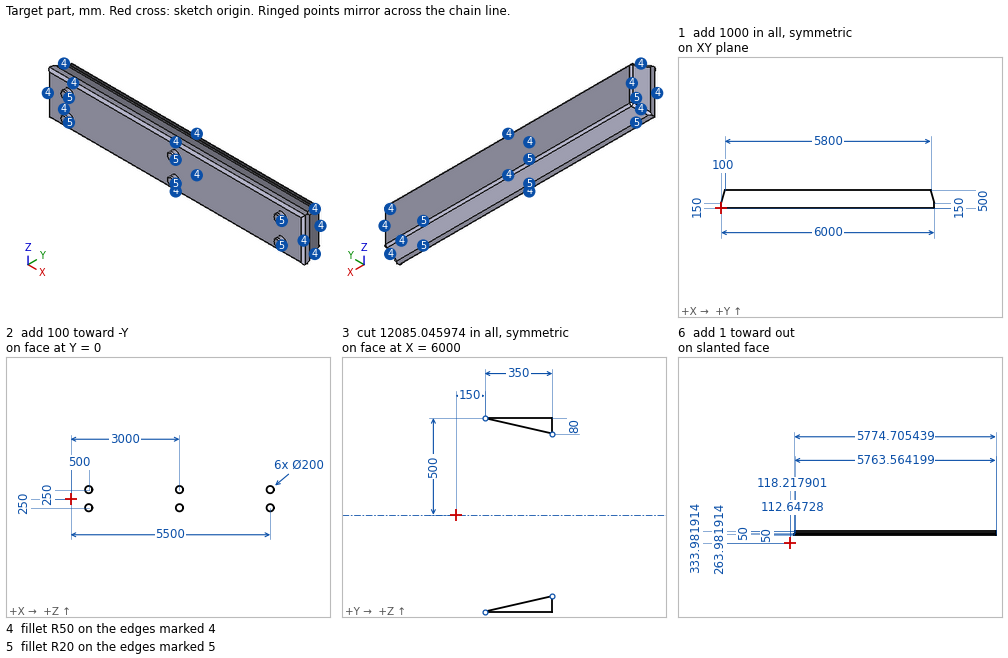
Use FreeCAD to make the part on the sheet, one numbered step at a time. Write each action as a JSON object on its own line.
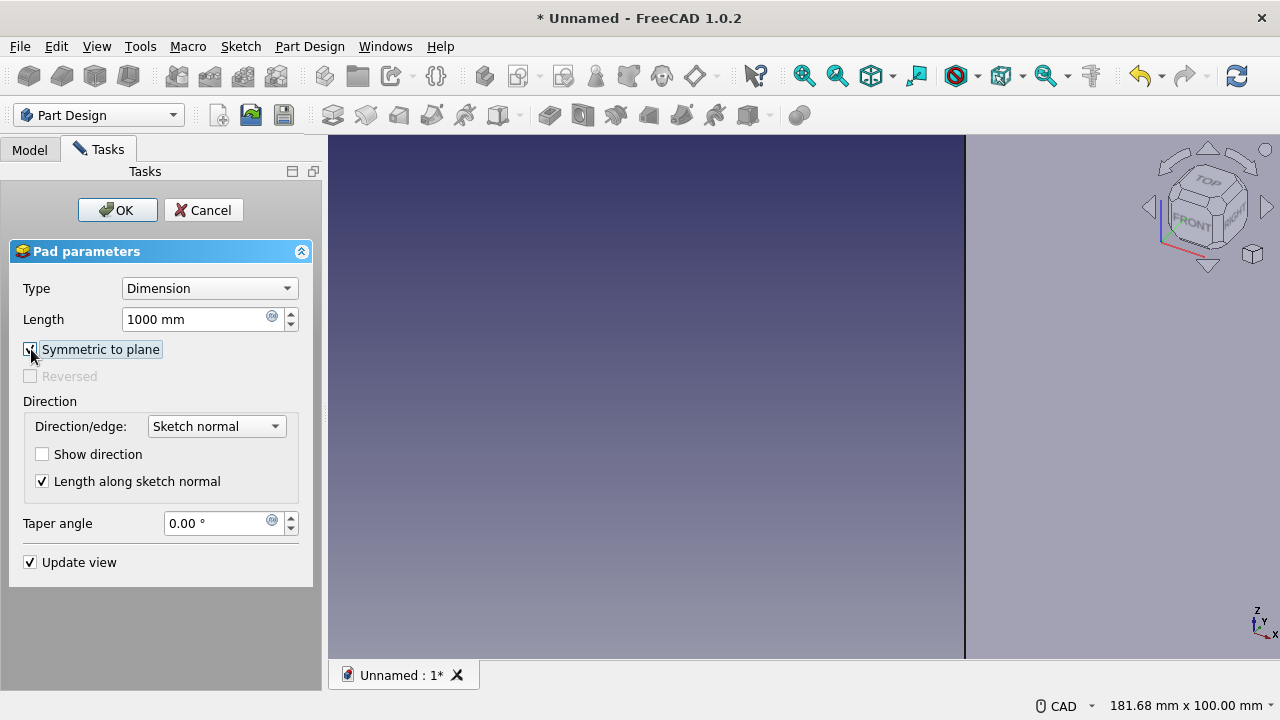
{"action": "left_click", "coordinate": [118, 210]}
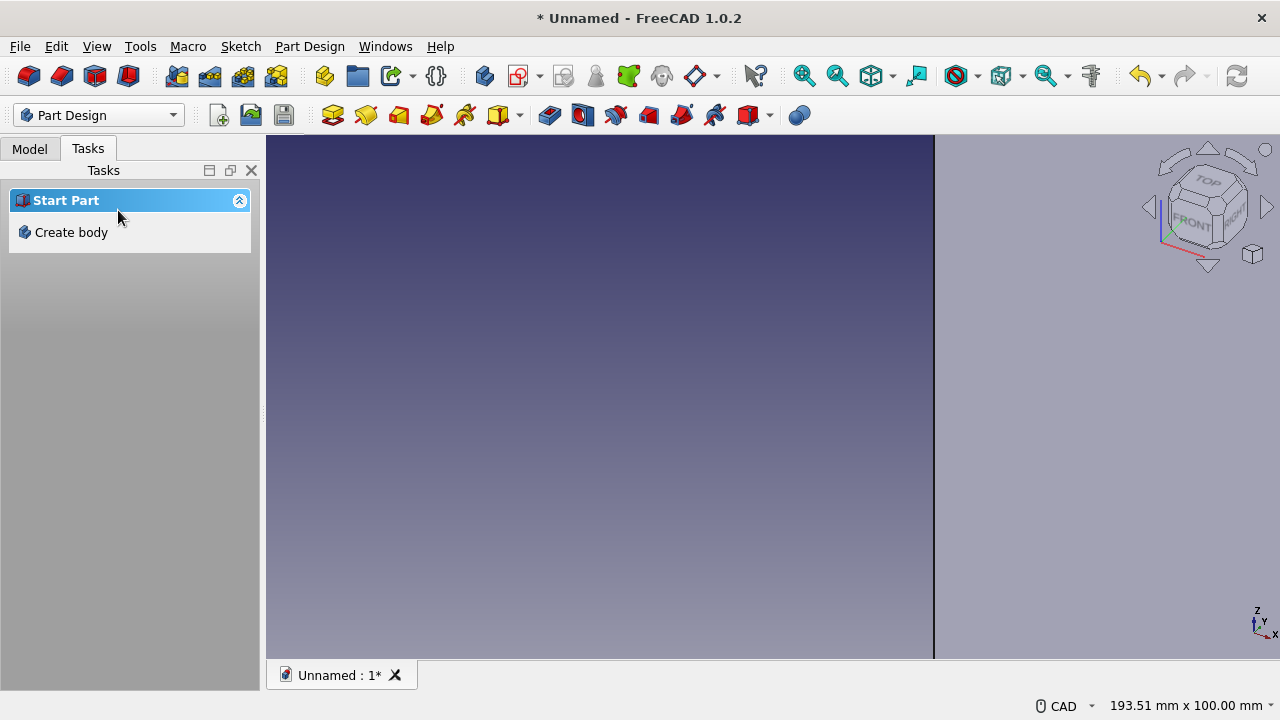
{"action": "left_click", "coordinate": [805, 76]}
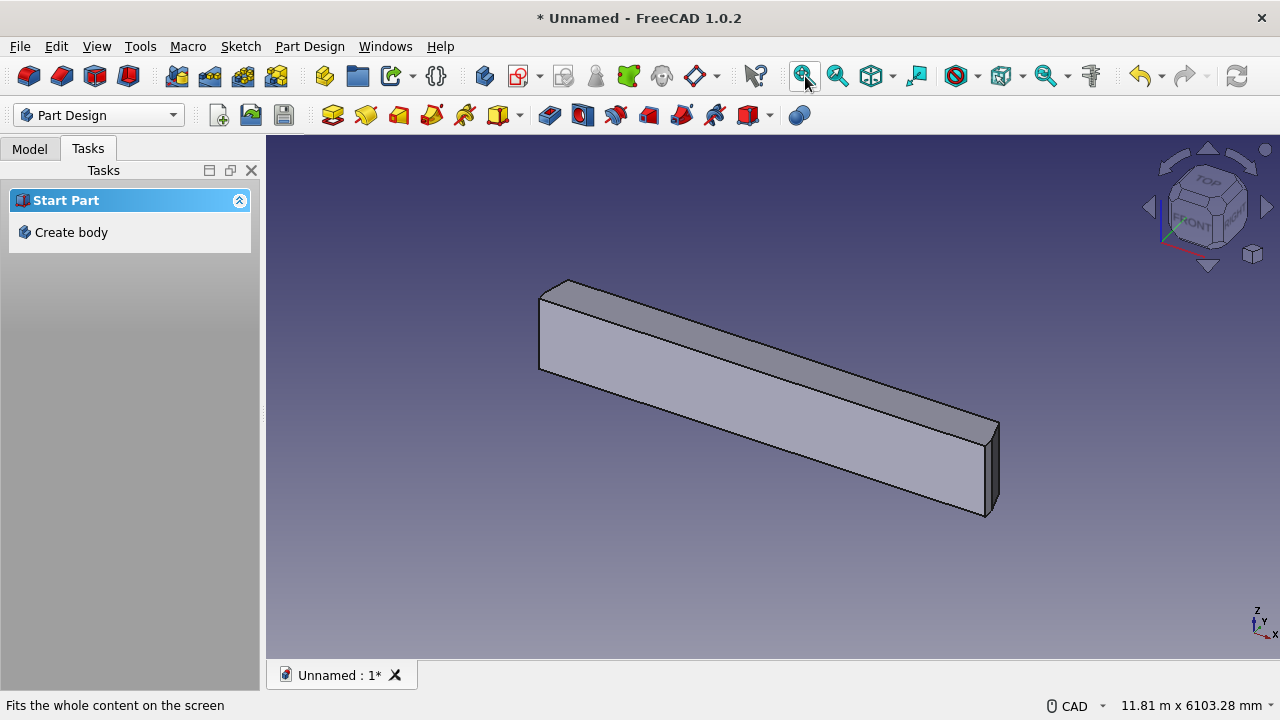
{"action": "left_click", "coordinate": [890, 449]}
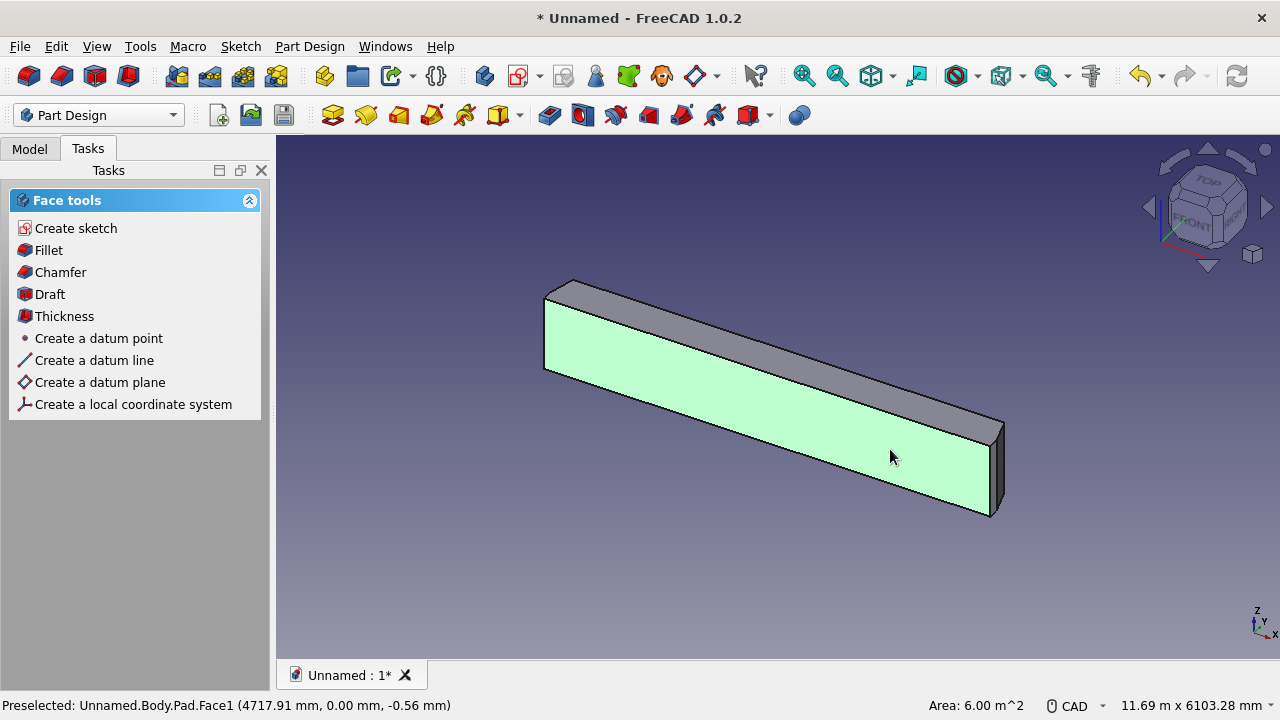
{"action": "left_click", "coordinate": [518, 76]}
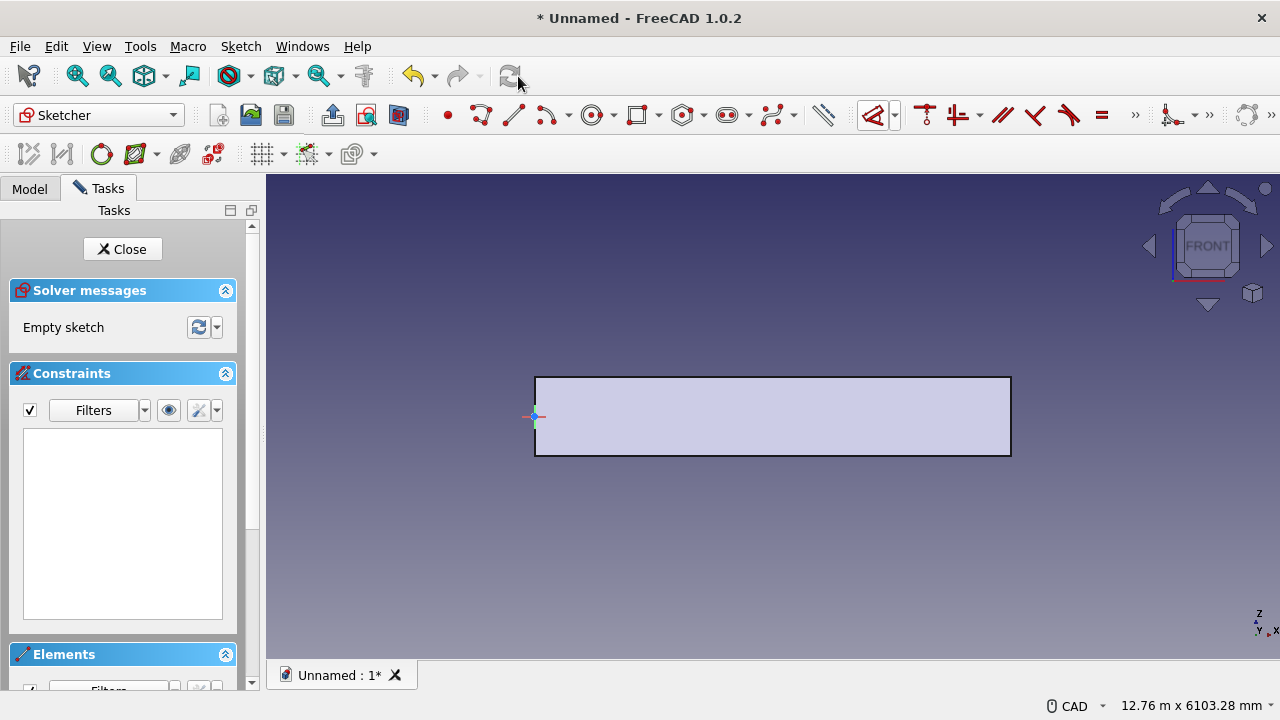
{"action": "left_click", "coordinate": [592, 116]}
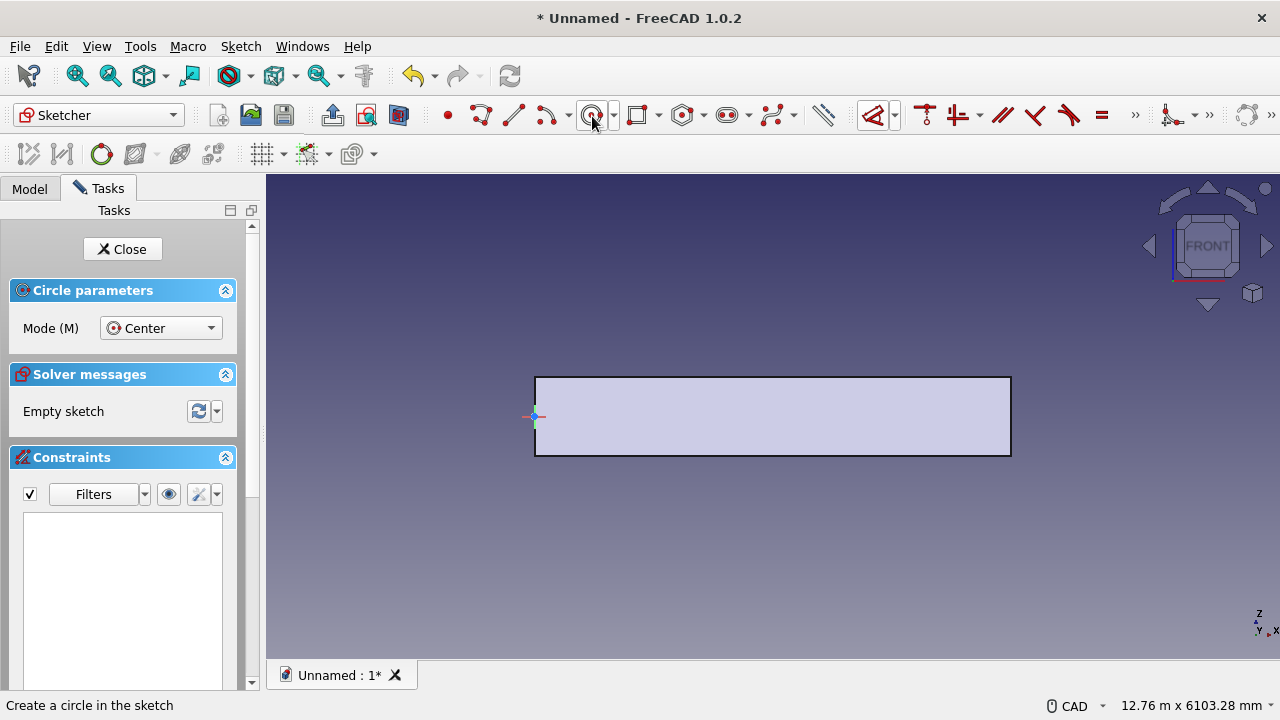
{"action": "scroll", "coordinate": [574, 397], "scroll_direction": "up", "scroll_amount": 6}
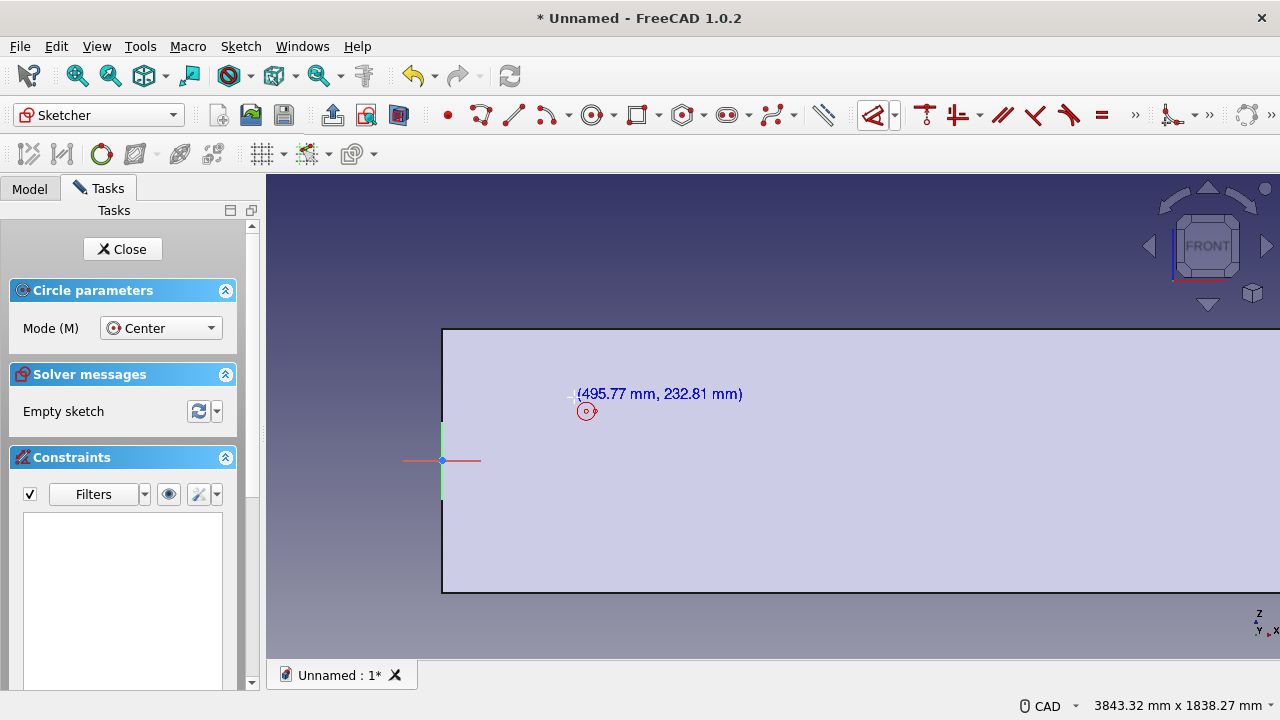
{"action": "left_click", "coordinate": [574, 395]}
{"action": "left_click", "coordinate": [593, 376]}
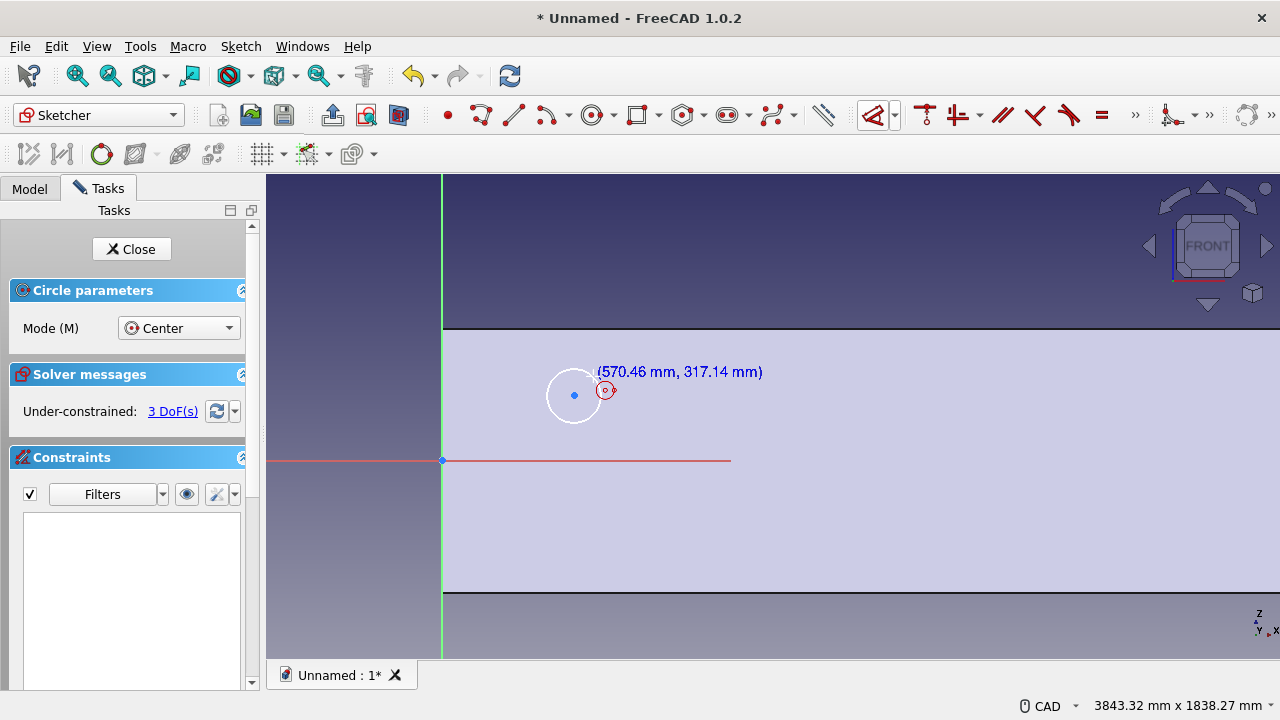
{"action": "left_click", "coordinate": [574, 527]}
{"action": "left_click", "coordinate": [593, 508]}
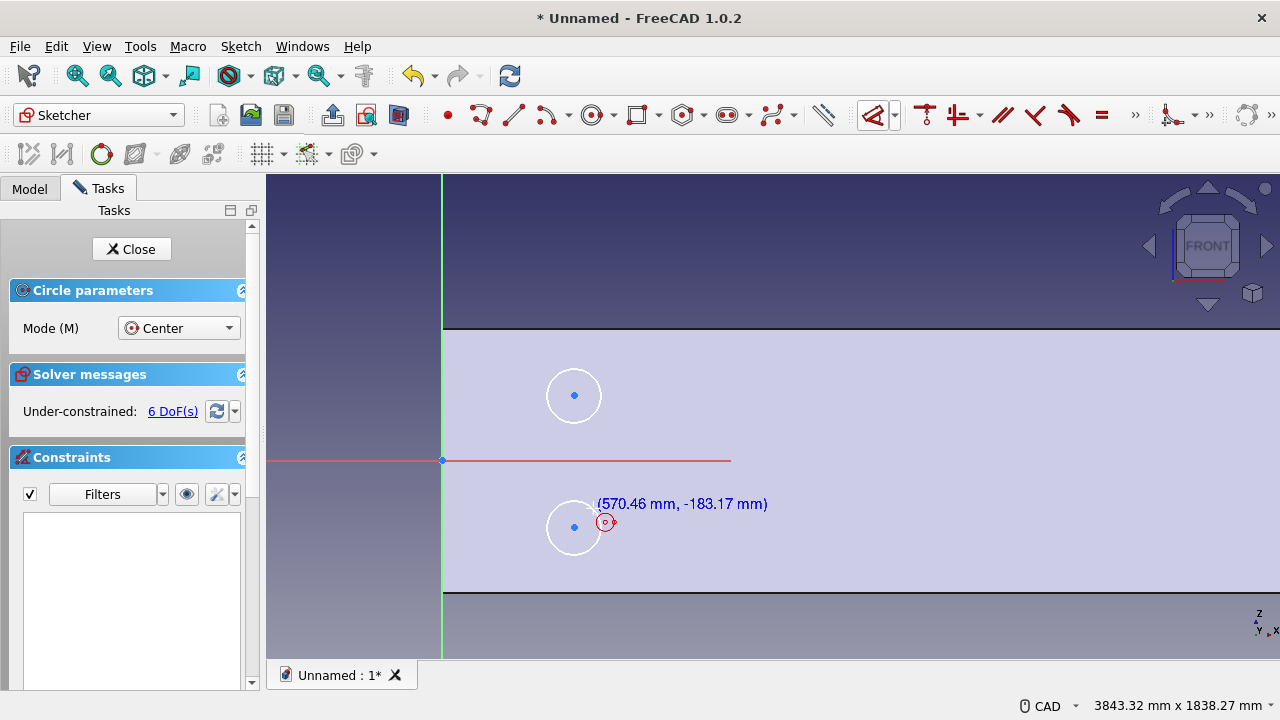
{"action": "scroll", "coordinate": [427, 391], "scroll_direction": "down", "scroll_amount": 5}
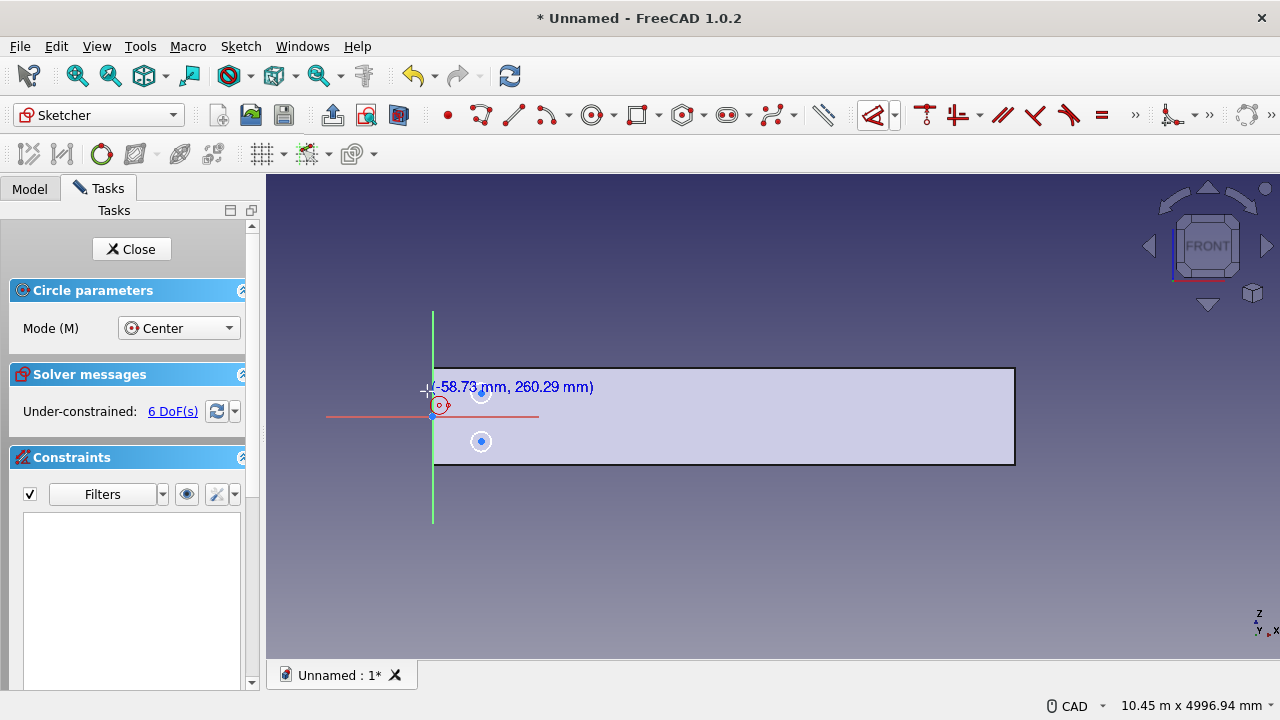
{"action": "scroll", "coordinate": [967, 441], "scroll_direction": "up", "scroll_amount": 5}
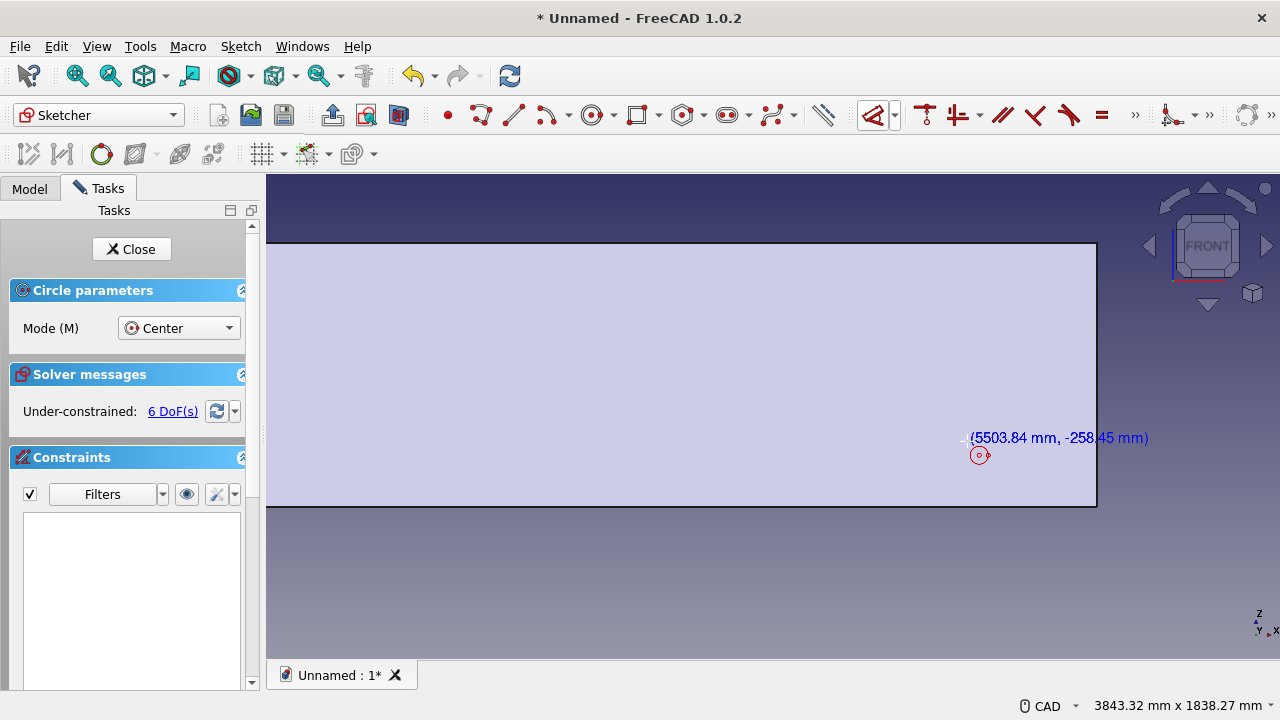
{"action": "left_click", "coordinate": [965, 441]}
{"action": "left_click", "coordinate": [983, 422]}